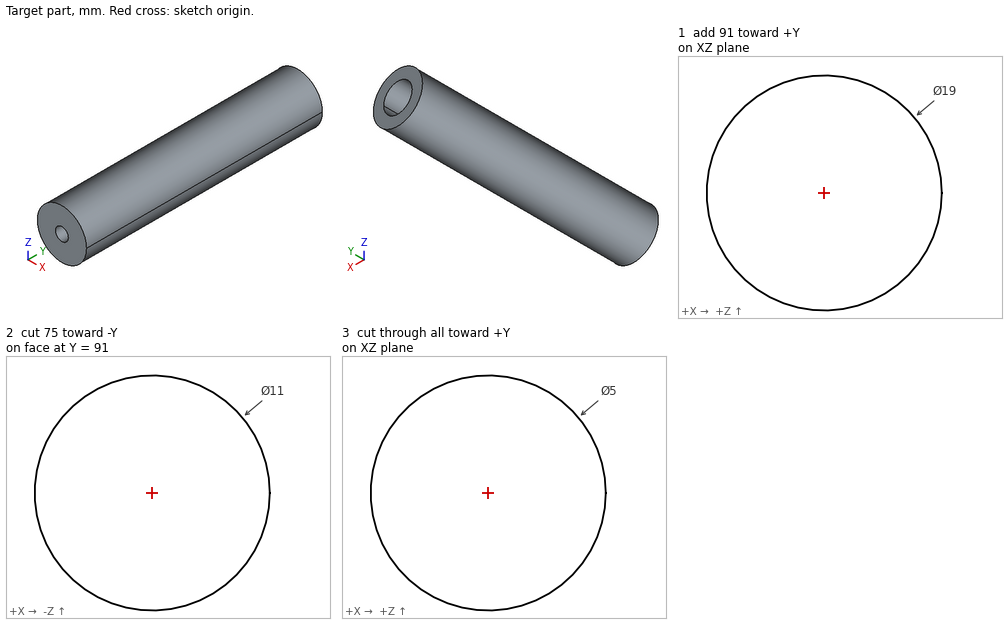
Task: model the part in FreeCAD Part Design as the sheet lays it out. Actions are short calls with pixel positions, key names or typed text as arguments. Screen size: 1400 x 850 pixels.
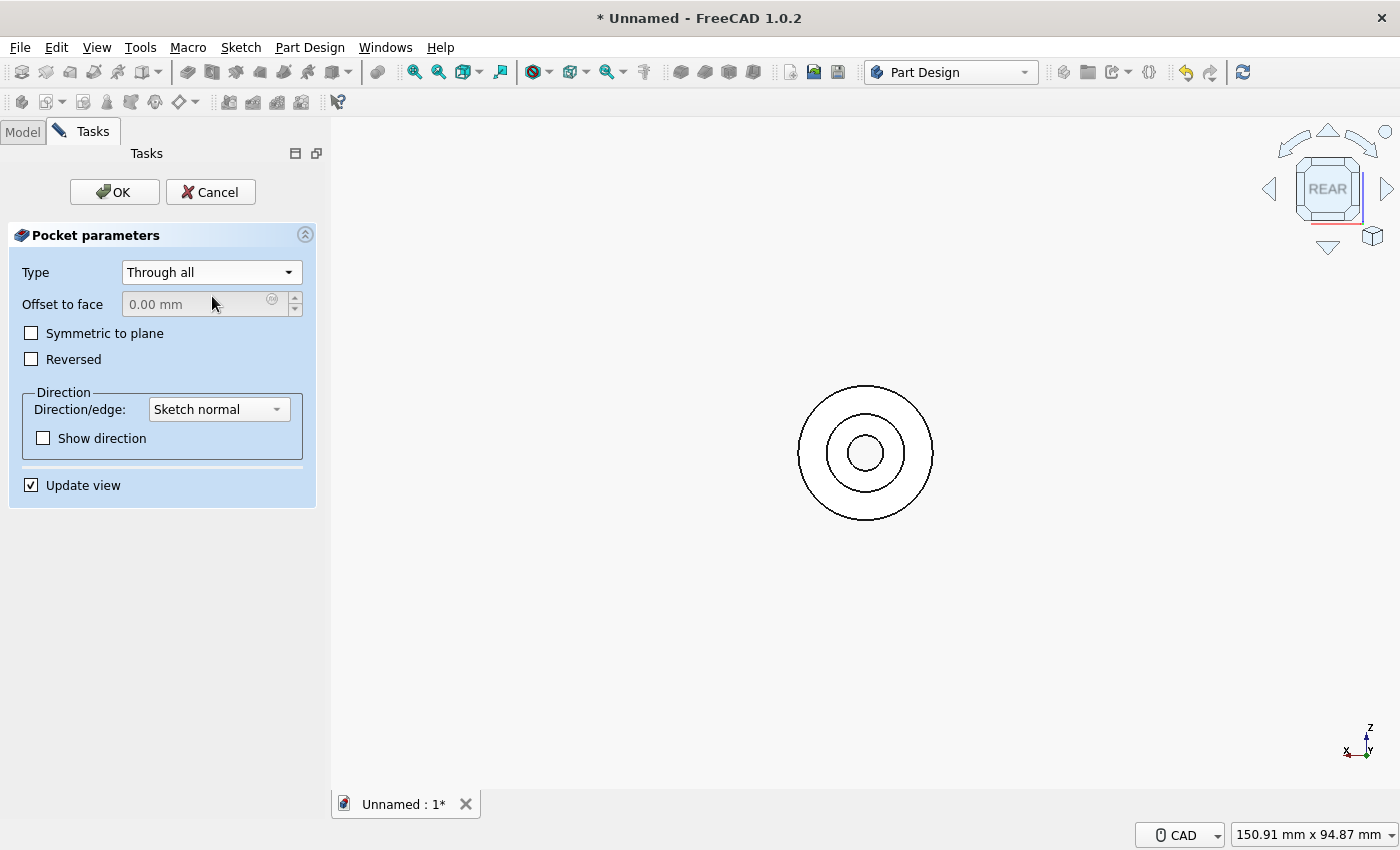
click(115, 192)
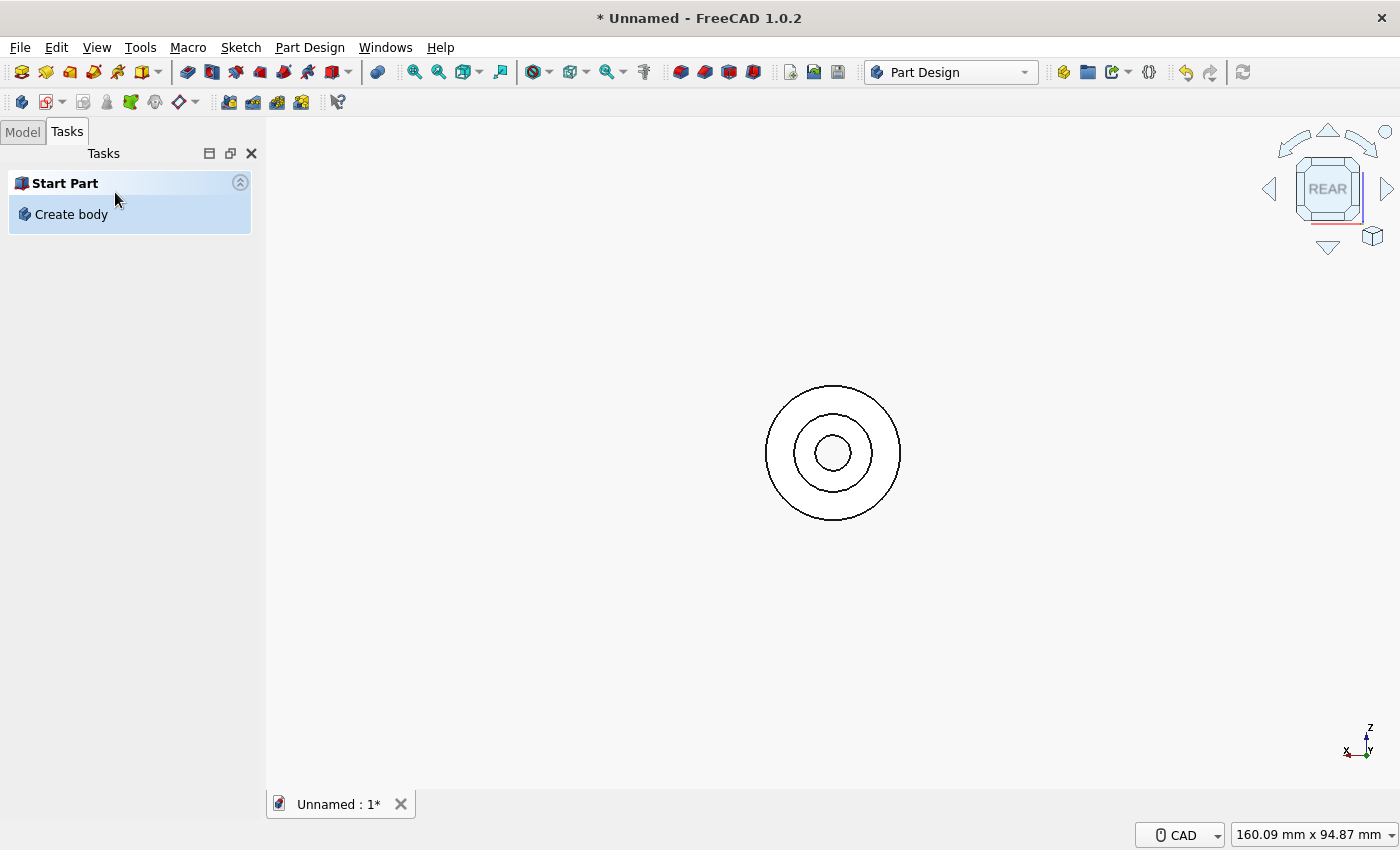
key(0)